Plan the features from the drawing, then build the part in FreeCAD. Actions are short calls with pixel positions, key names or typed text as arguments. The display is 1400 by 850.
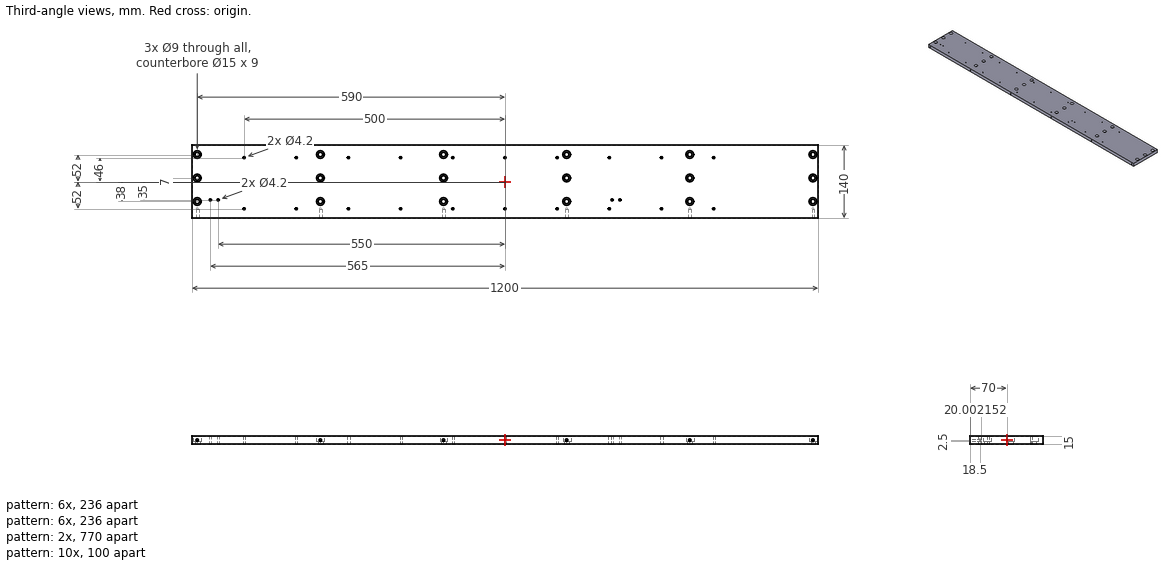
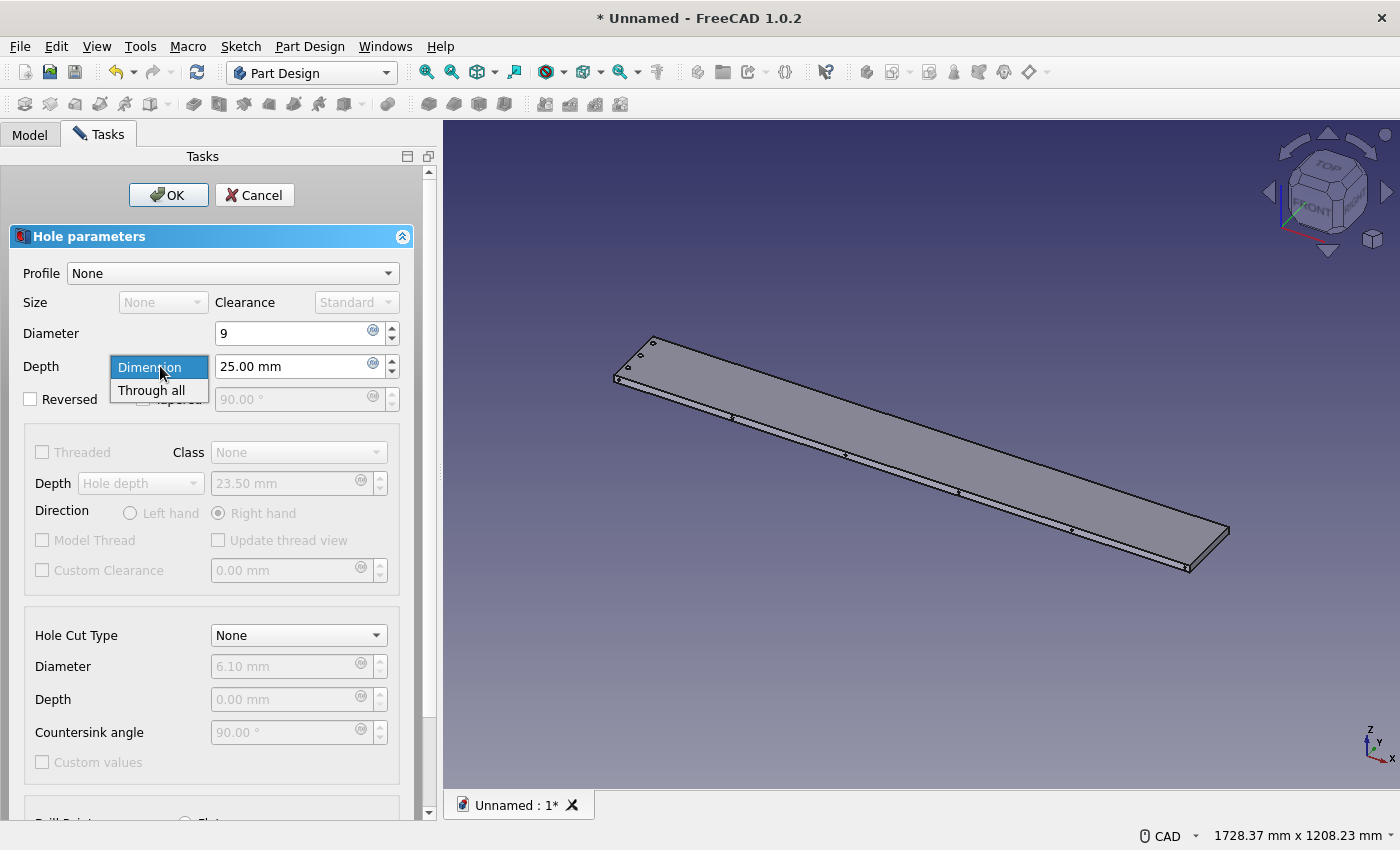
click(158, 390)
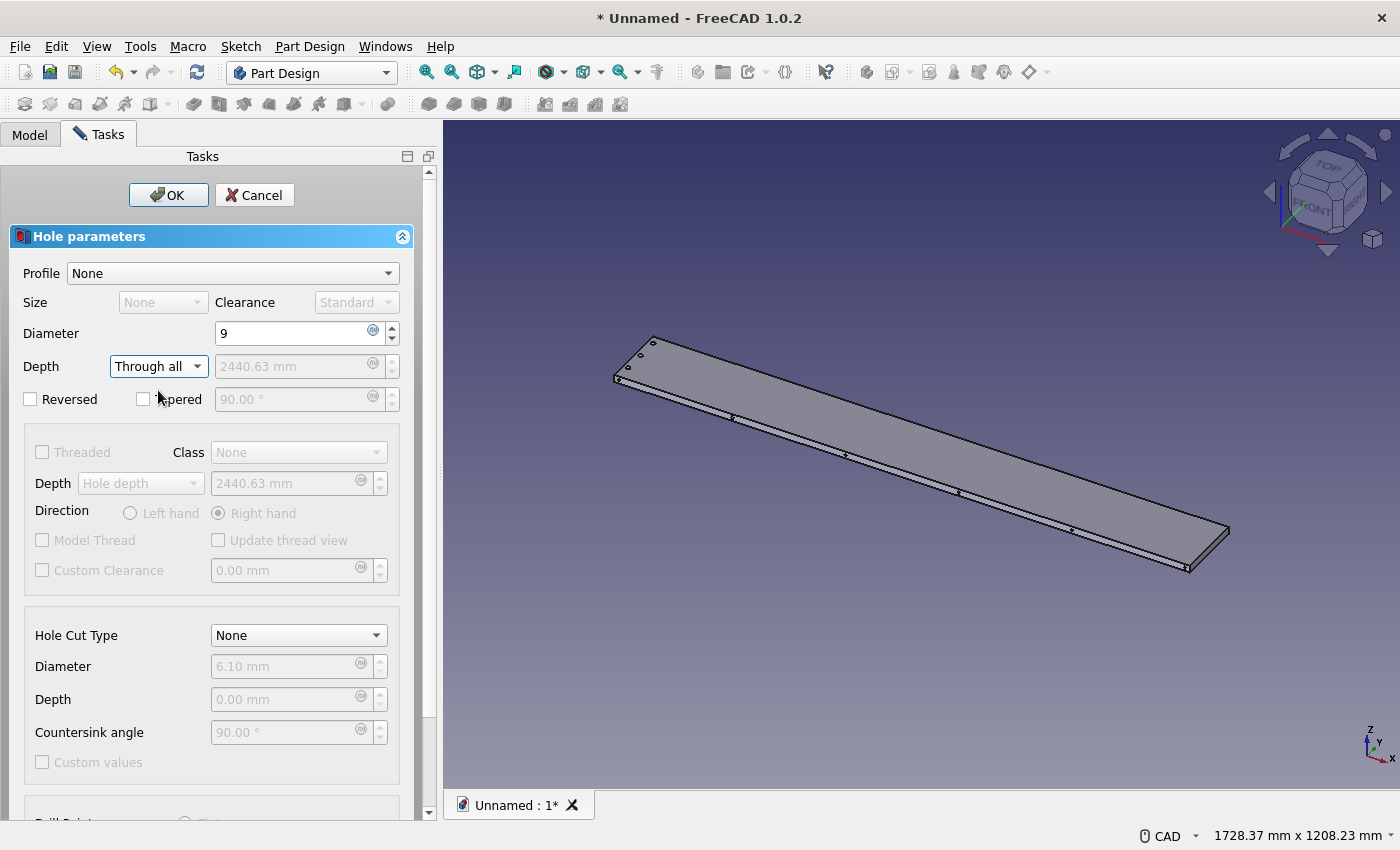
click(300, 636)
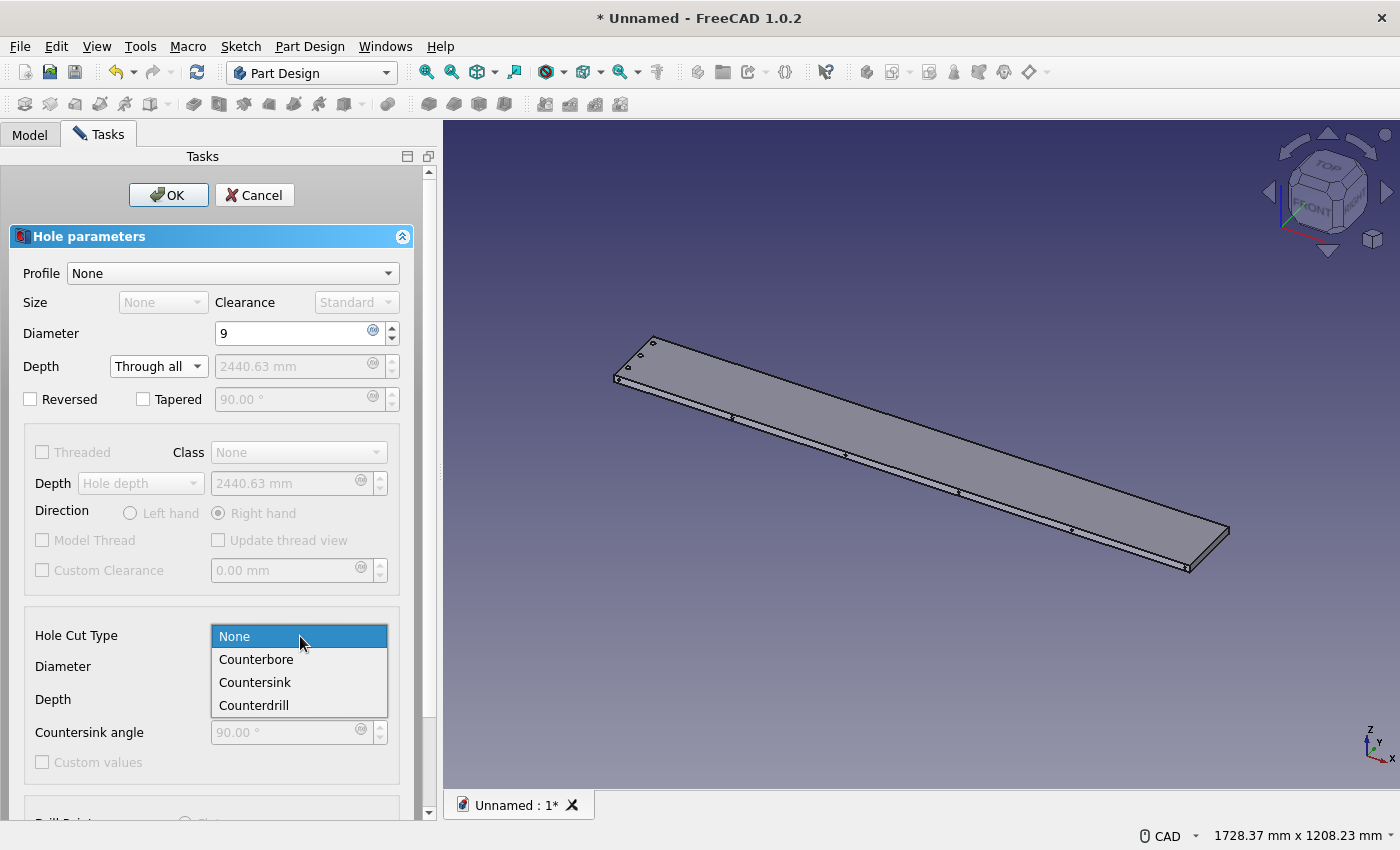
click(298, 660)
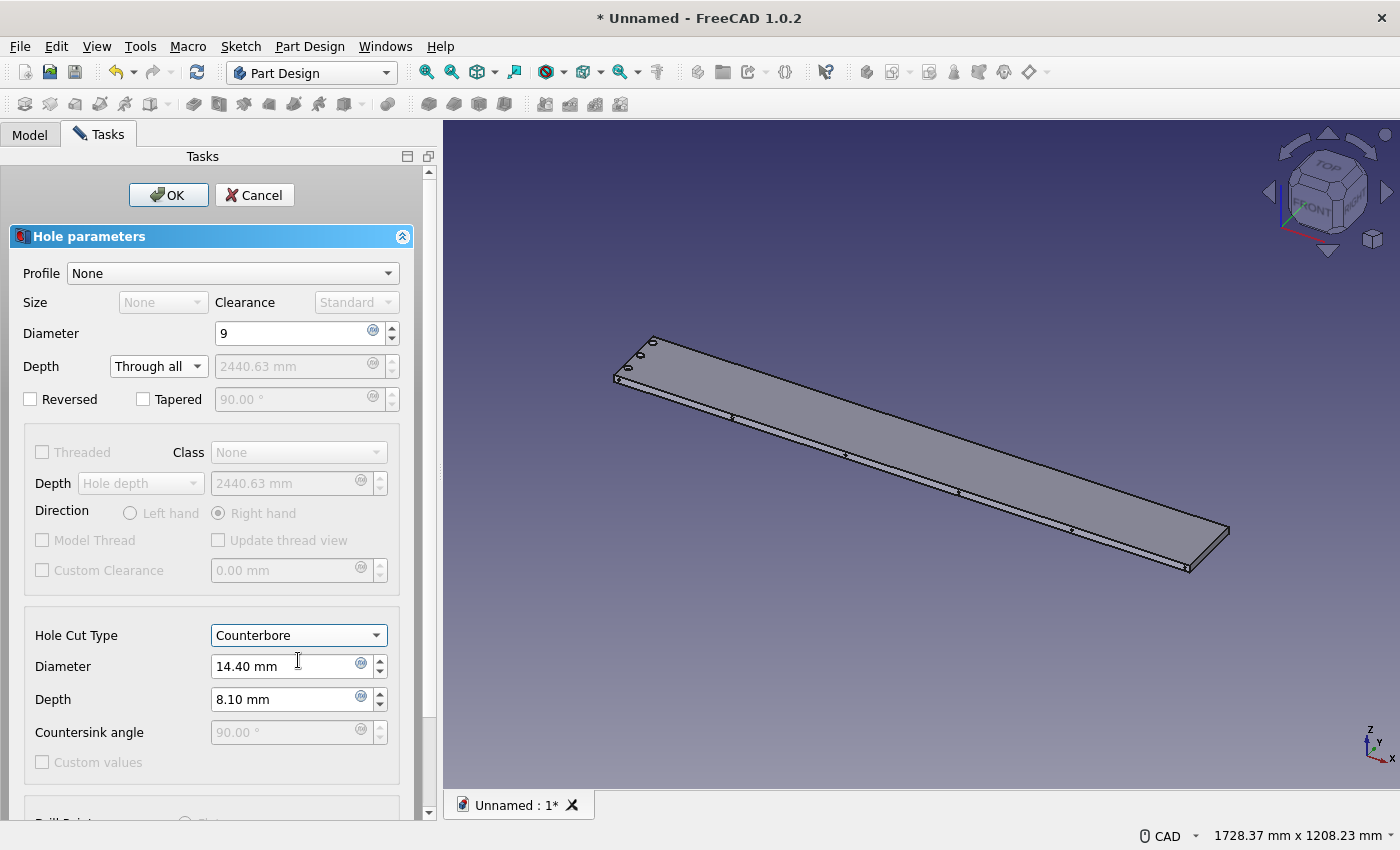
triple_click(292, 666)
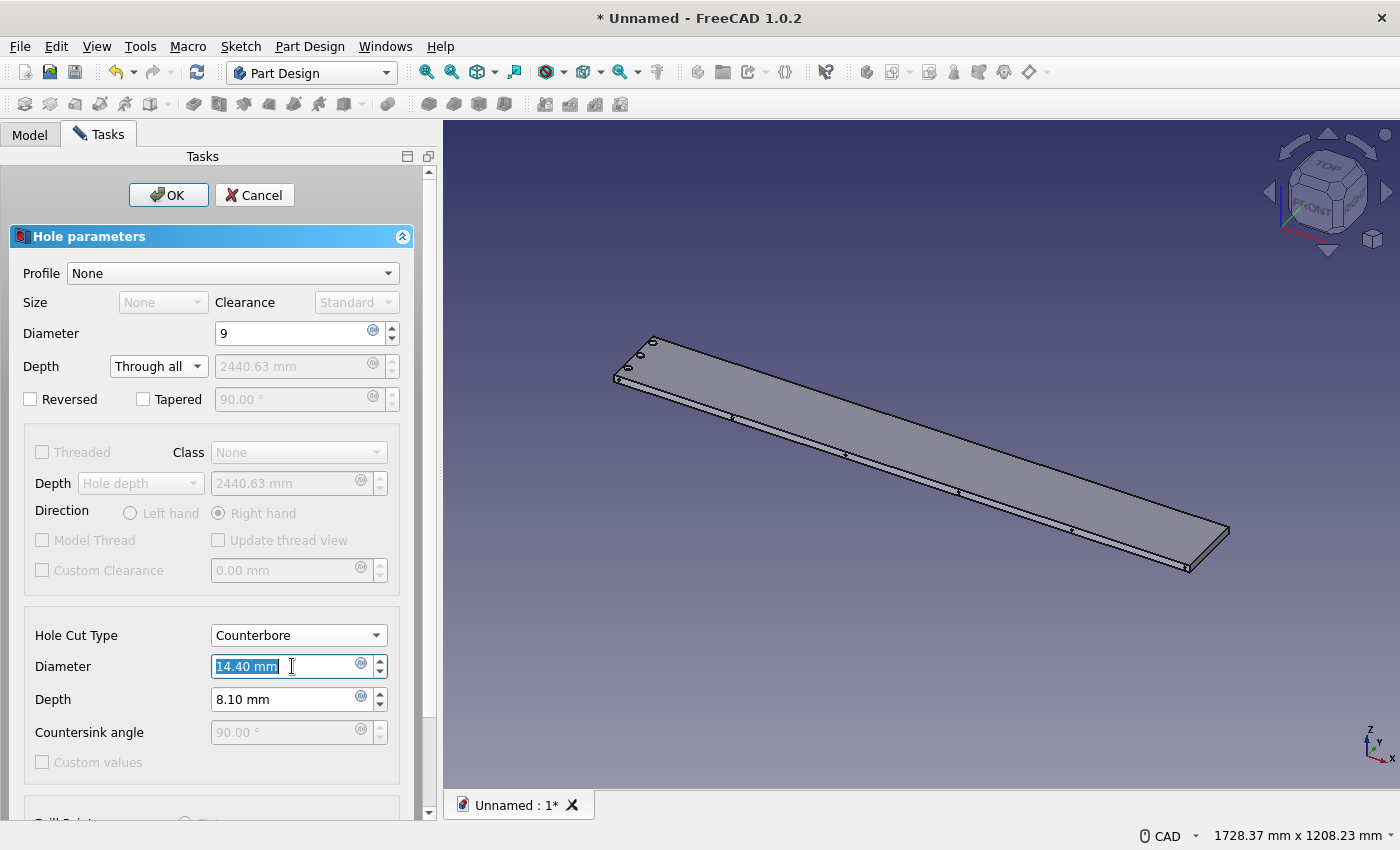
text(15)
key(Tab)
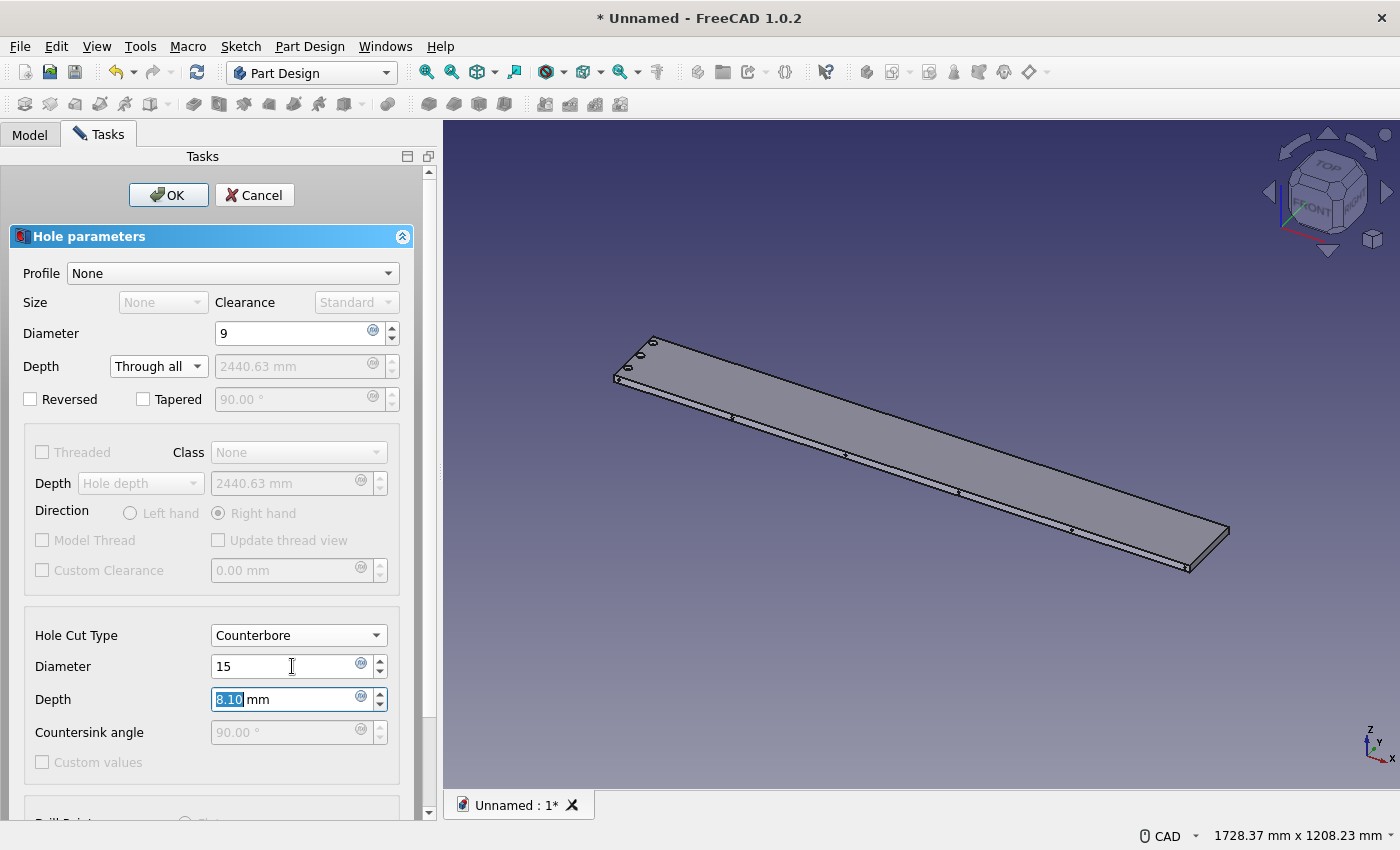
text(9)
key(Tab)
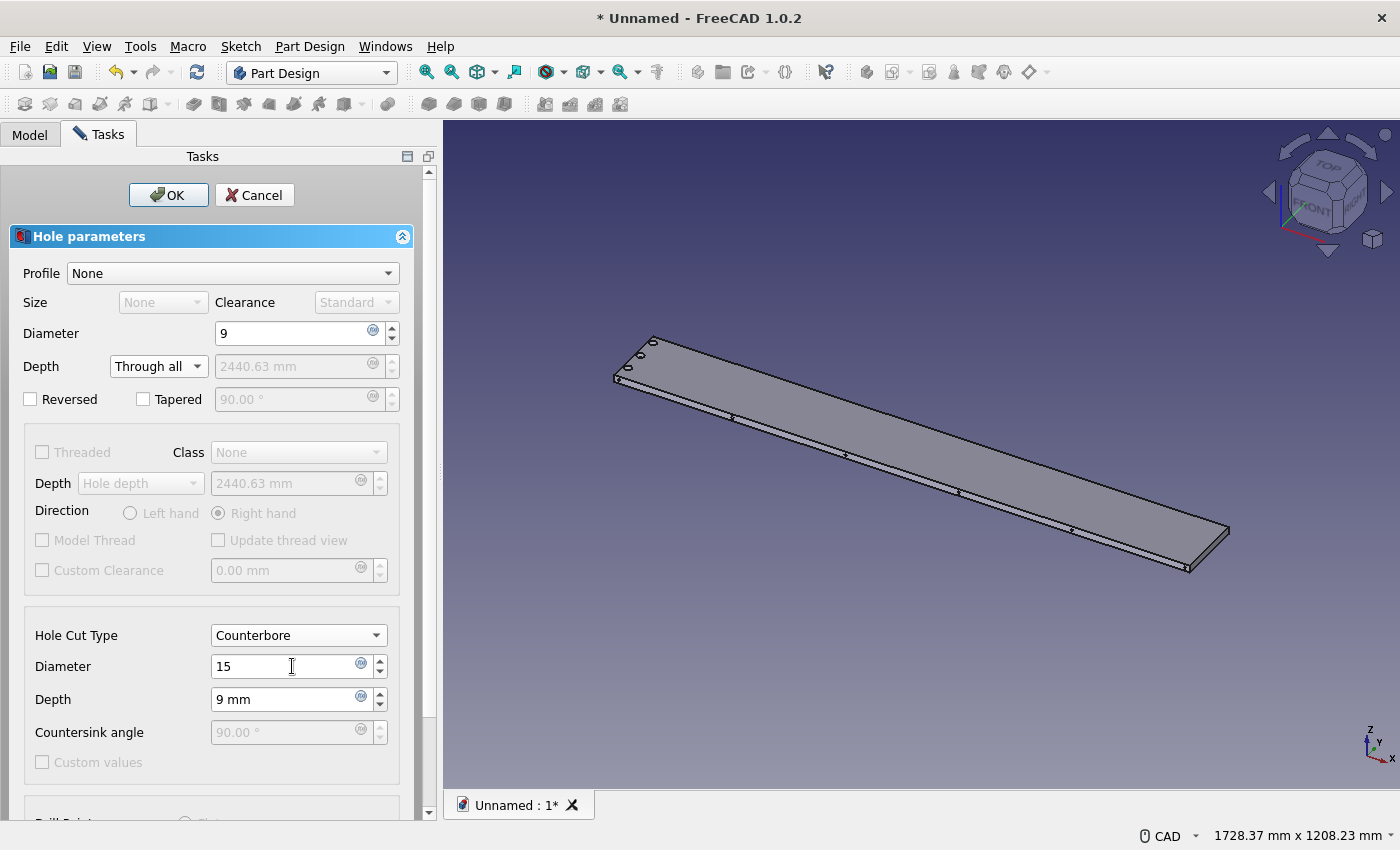
click(169, 195)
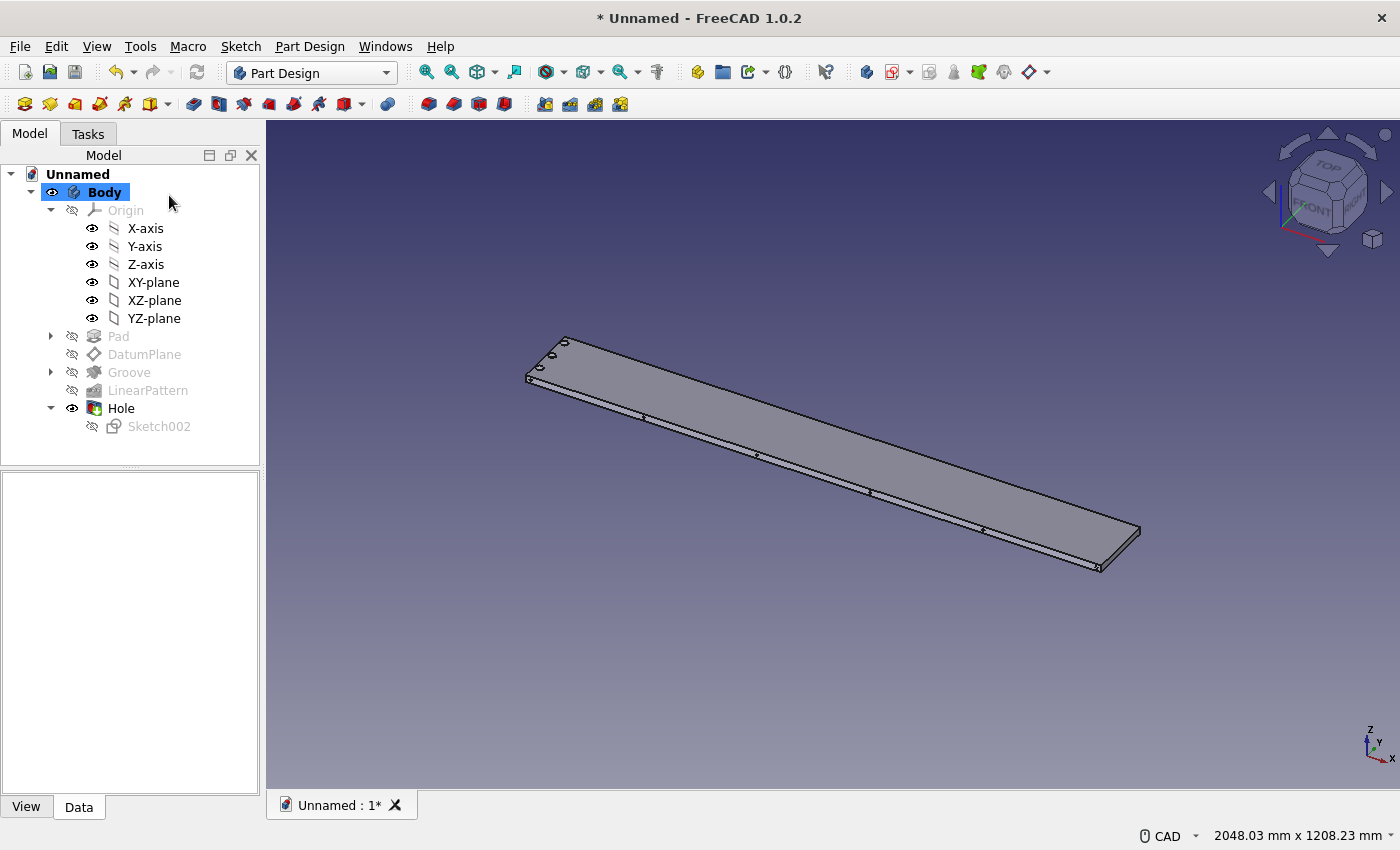
click(117, 408)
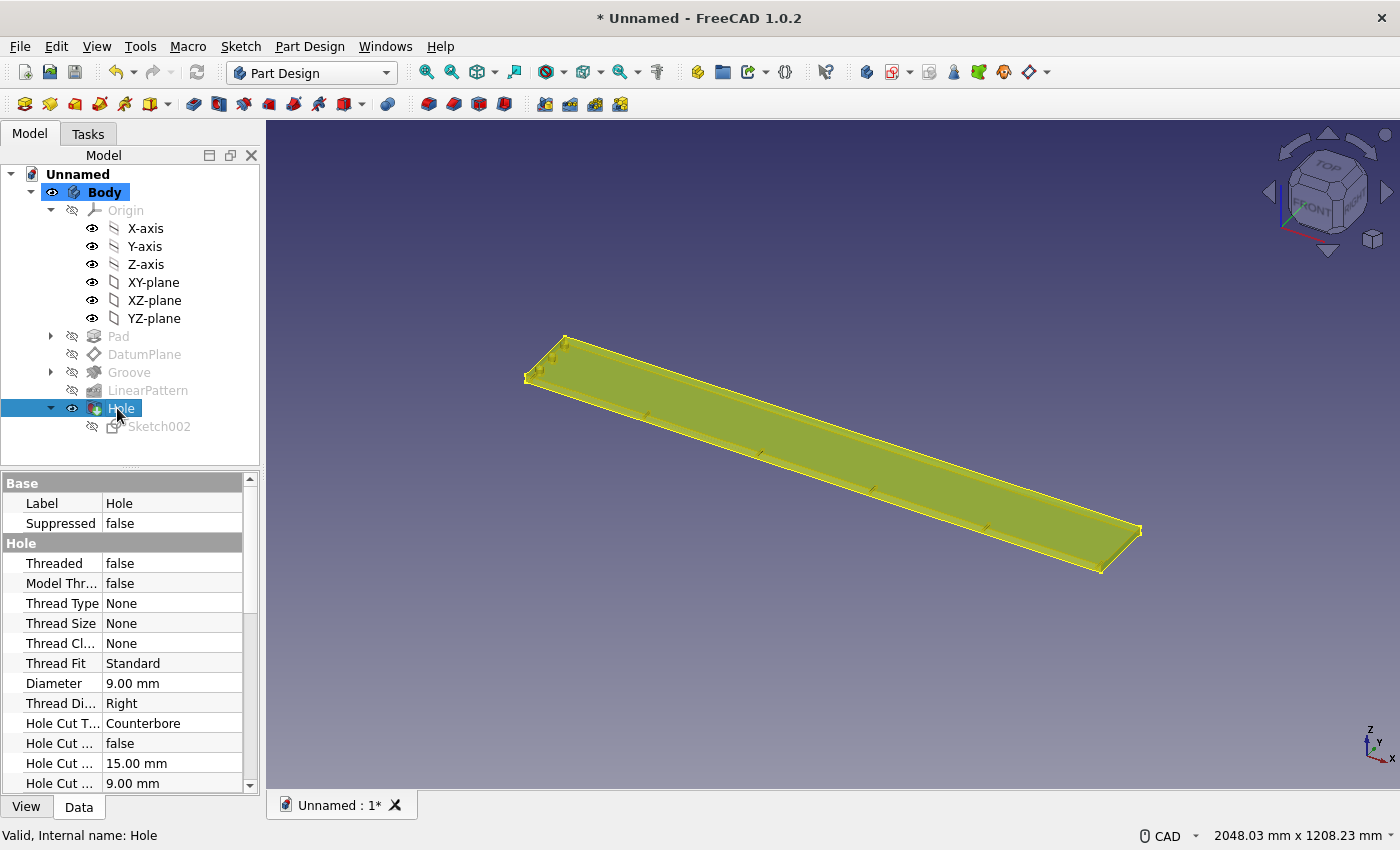
click(570, 104)